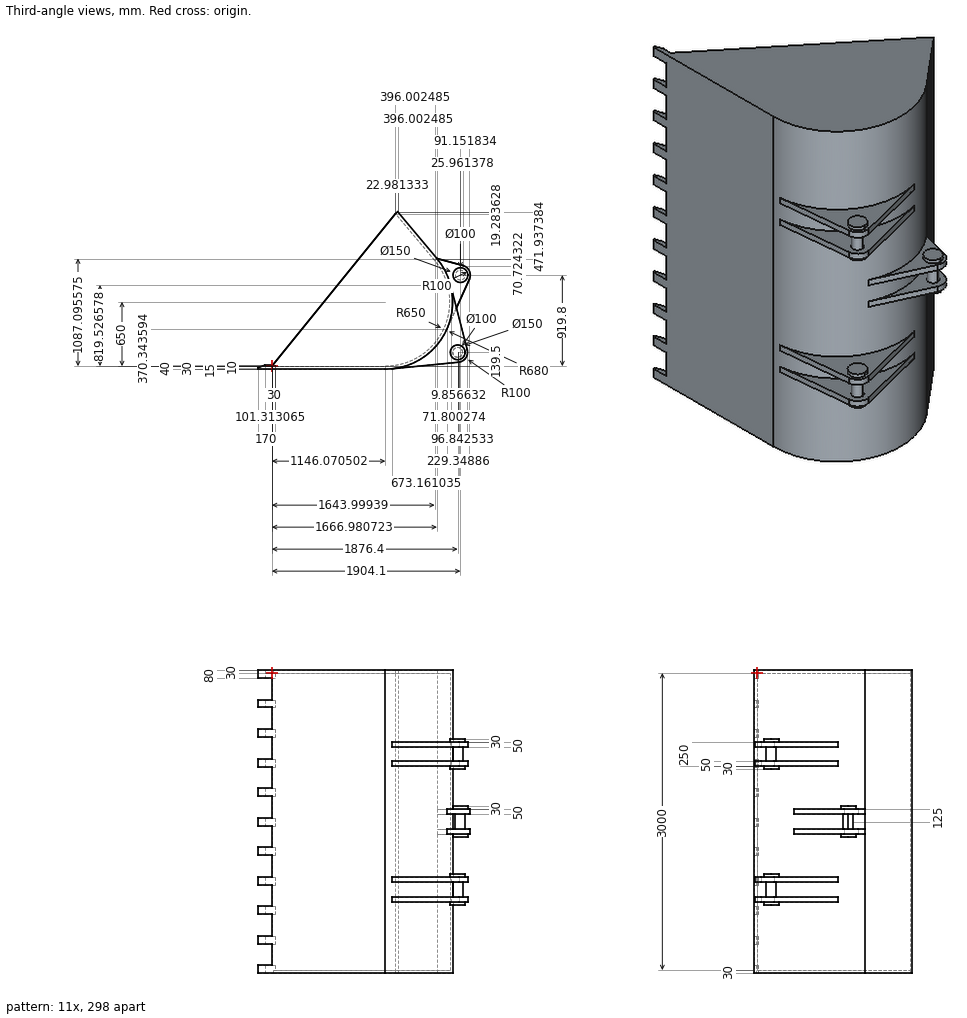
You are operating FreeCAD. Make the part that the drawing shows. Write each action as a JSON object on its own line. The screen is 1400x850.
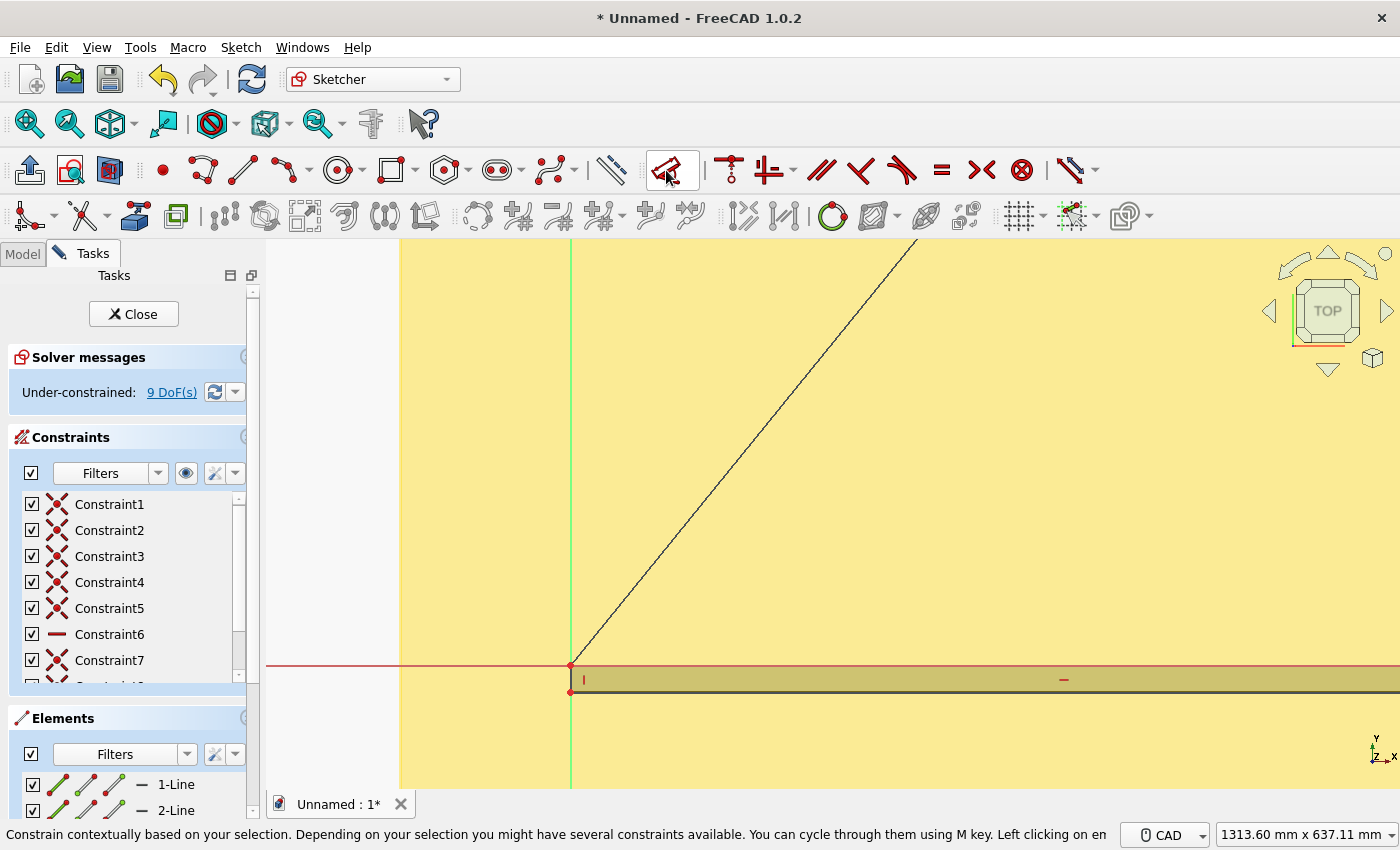
{"action": "scroll", "coordinate": [579, 680], "scroll_direction": "down", "scroll_amount": 7}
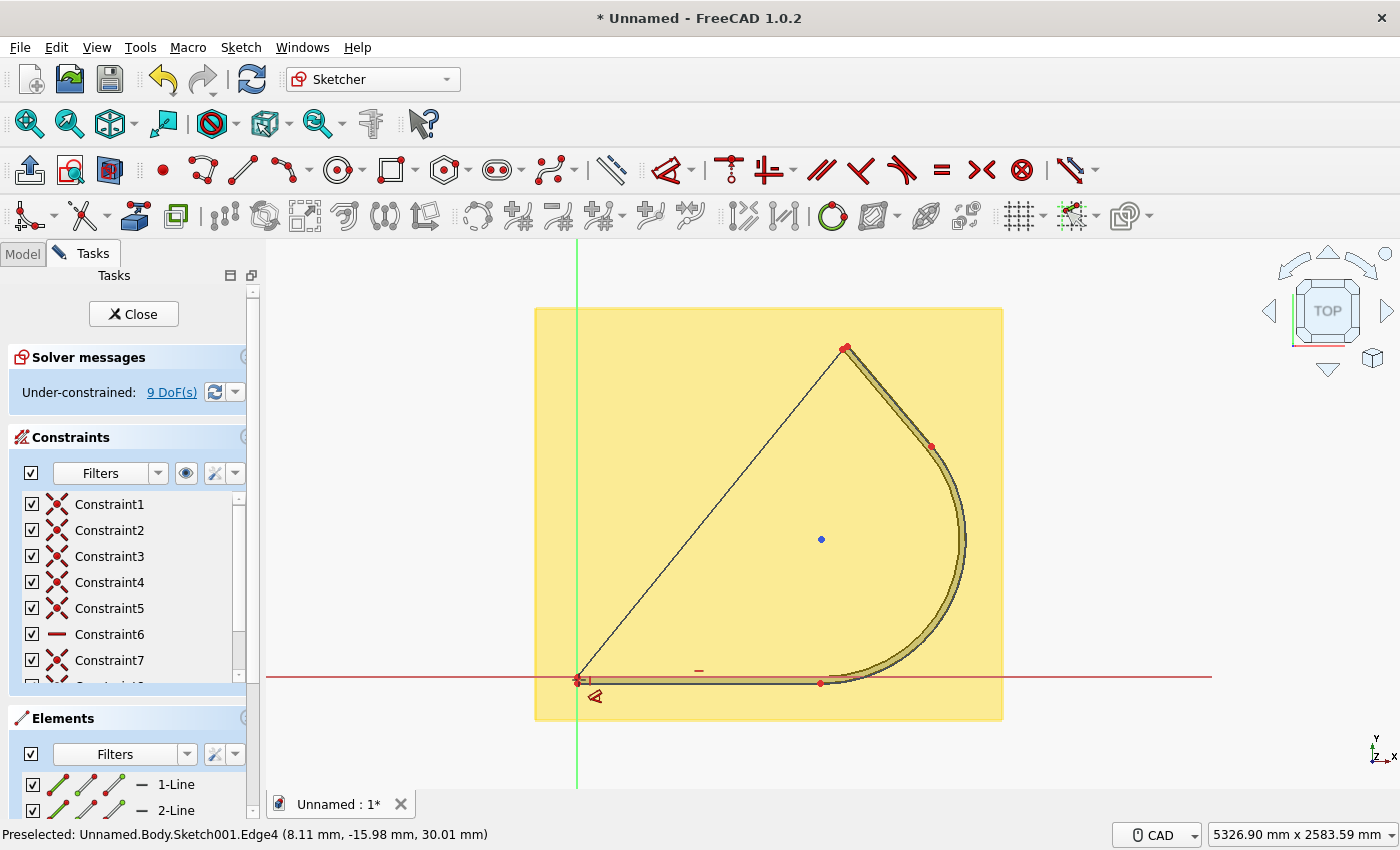
{"action": "left_click", "coordinate": [912, 652]}
{"action": "left_click", "coordinate": [853, 713]}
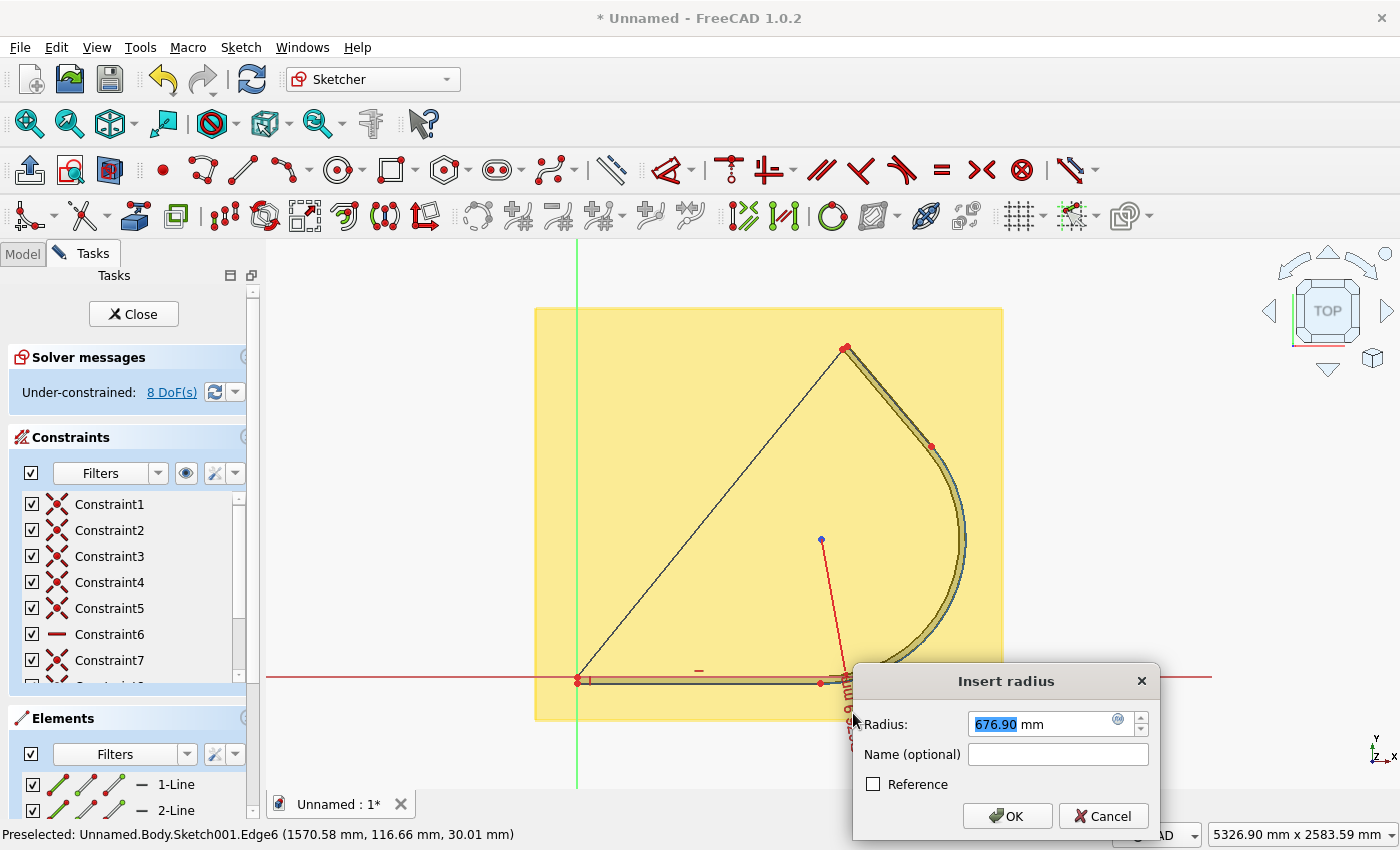
{"action": "type", "text": "680"}
{"action": "key", "text": "Return"}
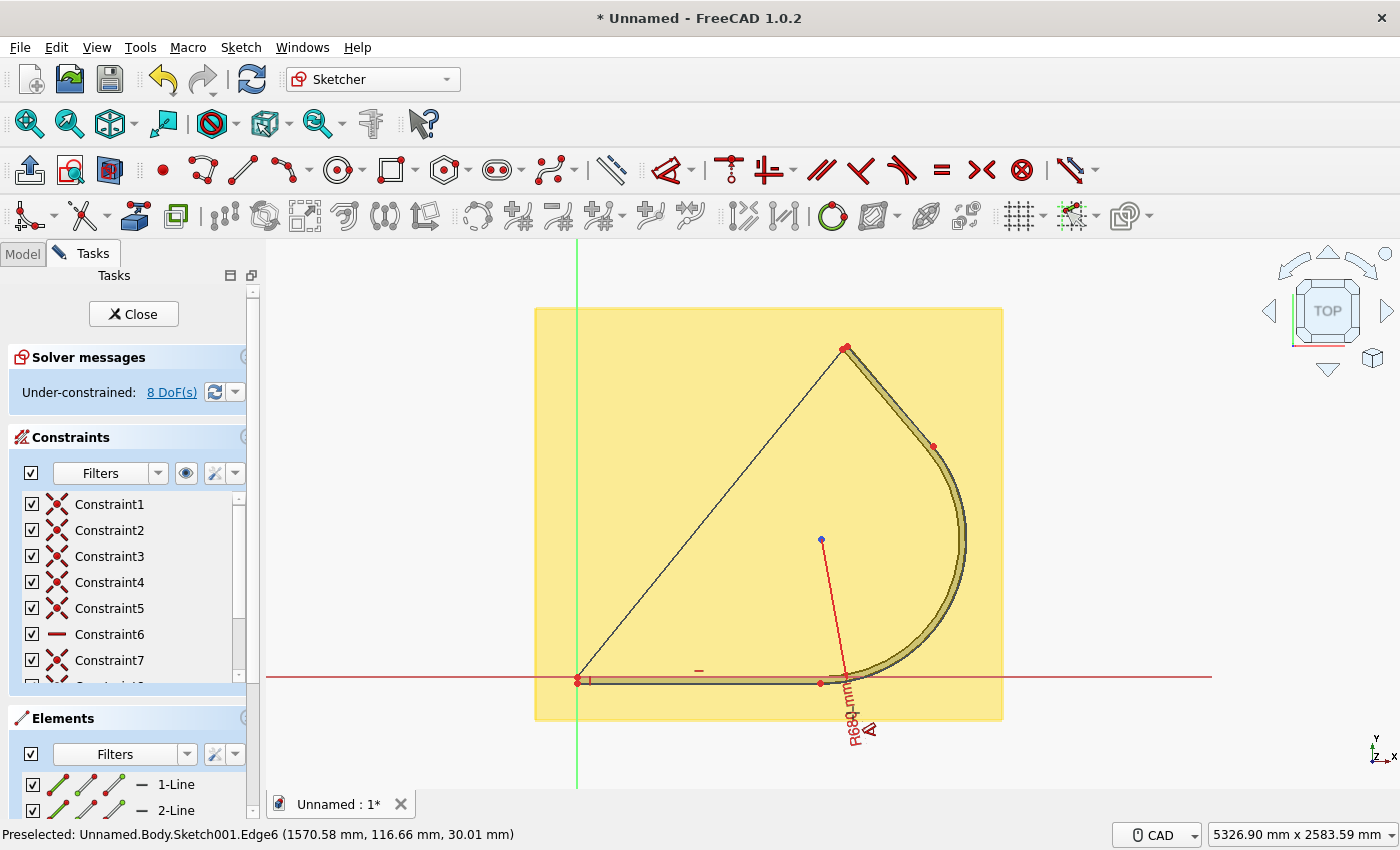
{"action": "scroll", "coordinate": [577, 680], "scroll_direction": "up", "scroll_amount": 10}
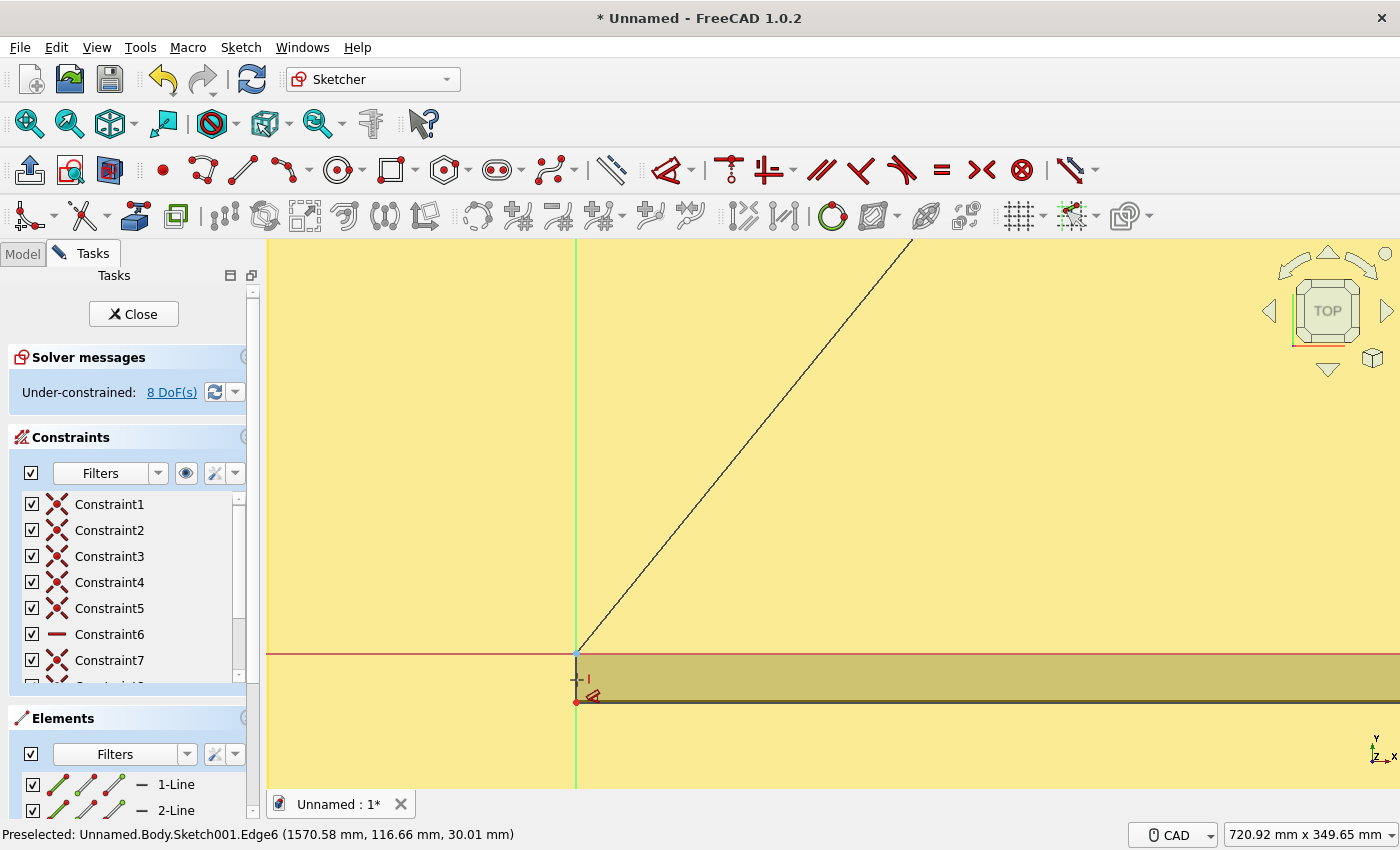
{"action": "left_click", "coordinate": [576, 678]}
{"action": "left_click", "coordinate": [542, 678]}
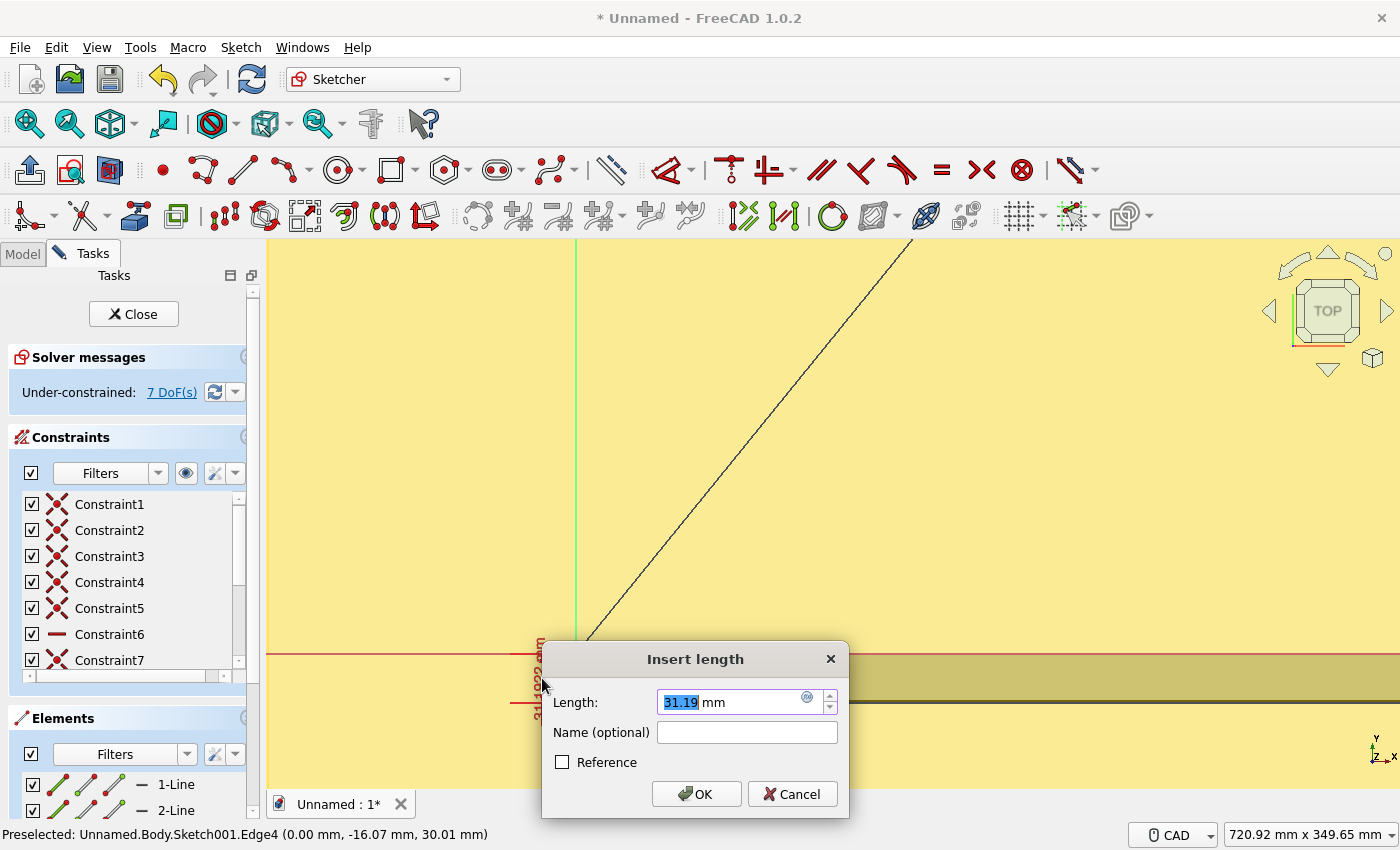
{"action": "type", "text": "30"}
{"action": "key", "text": "Return"}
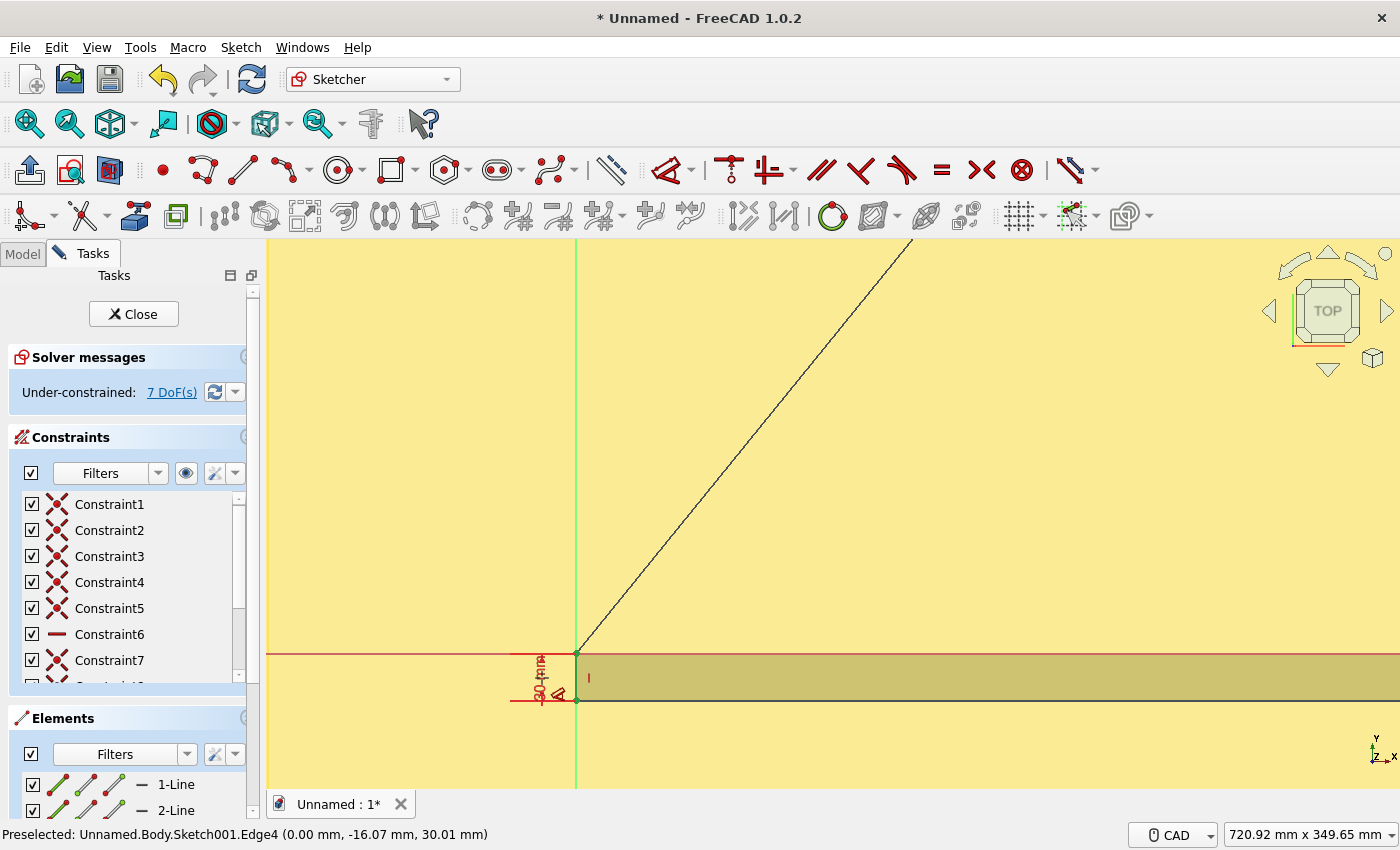
{"action": "scroll", "coordinate": [577, 680], "scroll_direction": "down", "scroll_amount": 10}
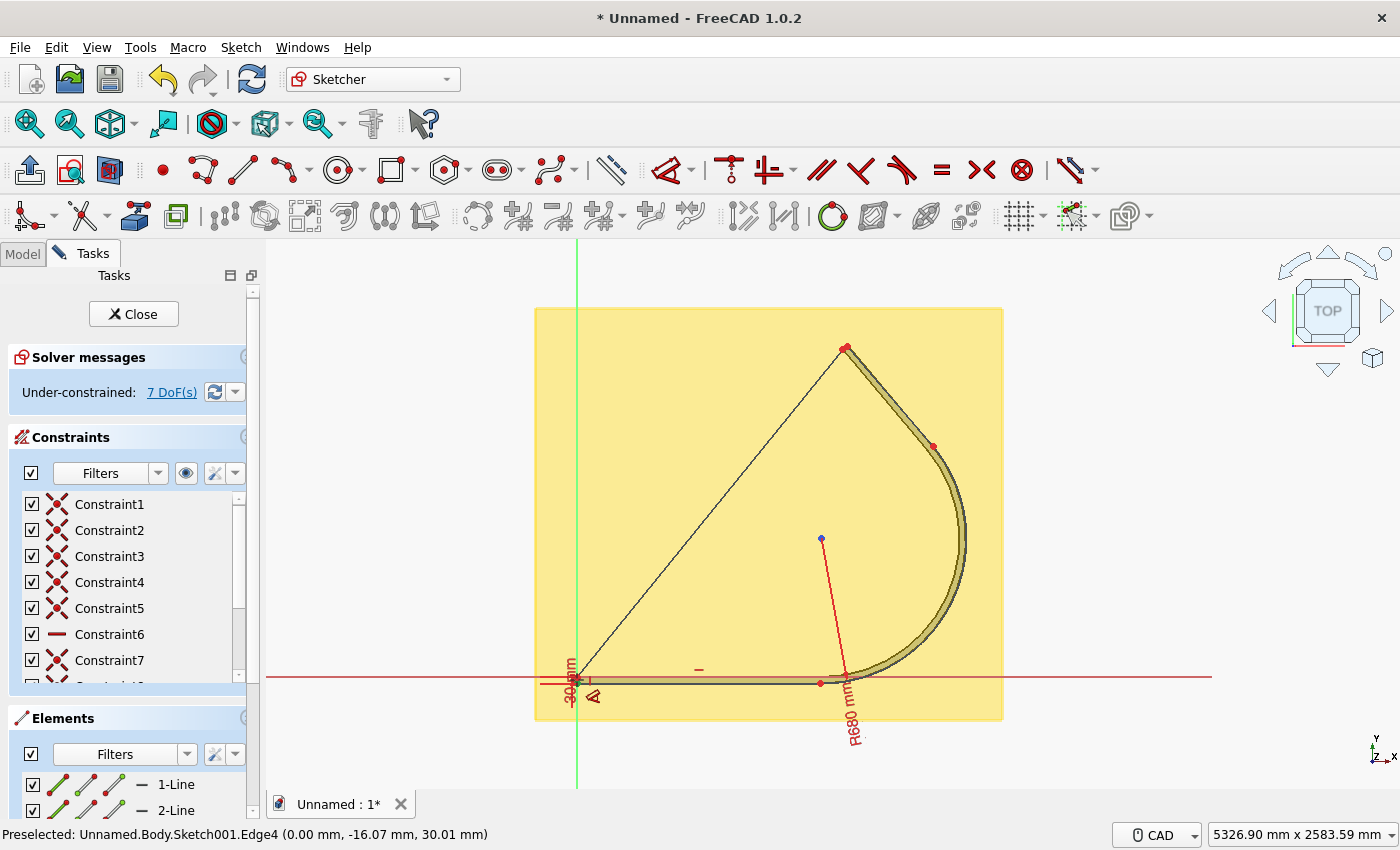
{"action": "scroll", "coordinate": [846, 348], "scroll_direction": "up", "scroll_amount": 11}